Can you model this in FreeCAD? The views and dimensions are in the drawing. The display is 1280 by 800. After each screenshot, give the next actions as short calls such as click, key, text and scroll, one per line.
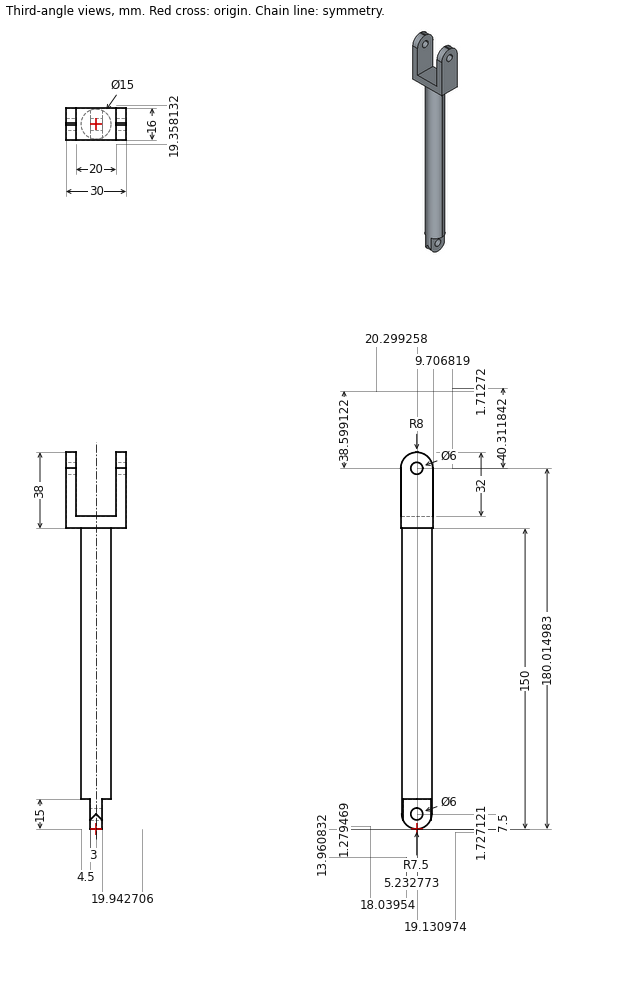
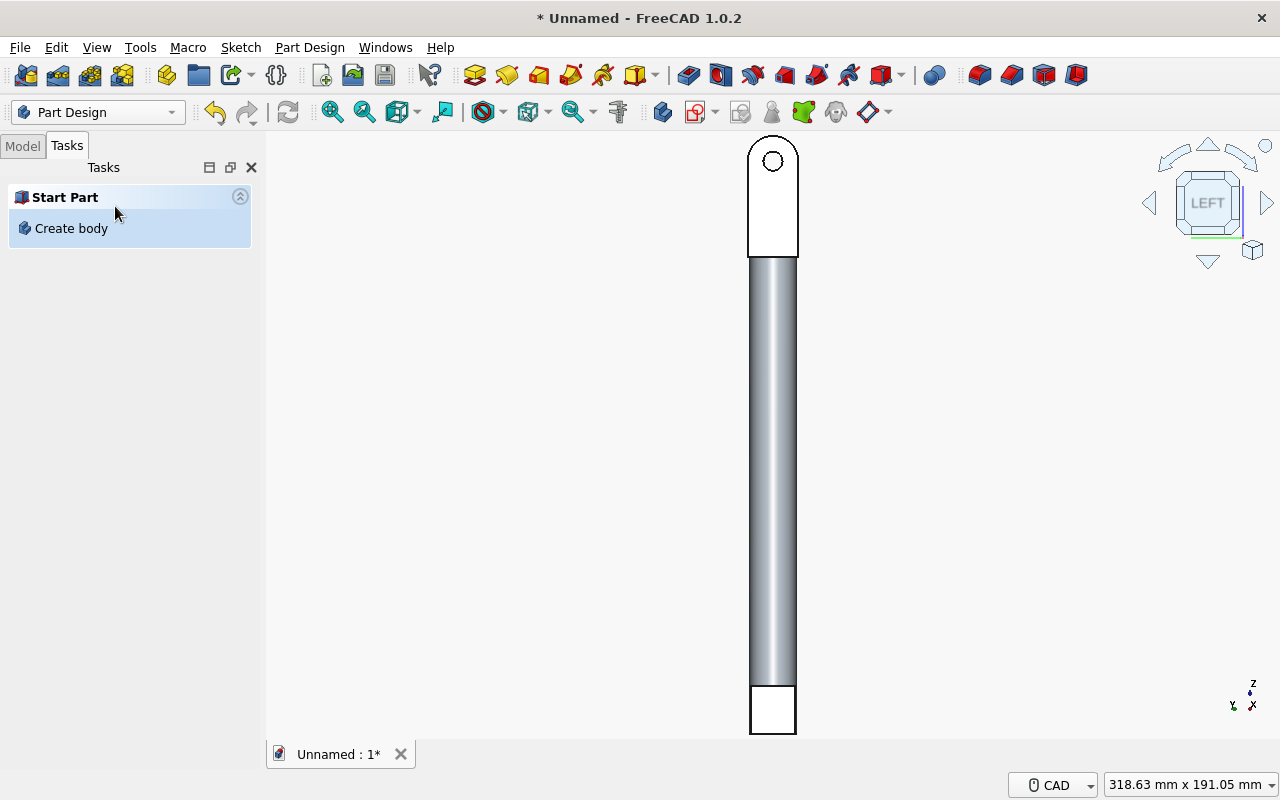
click(773, 709)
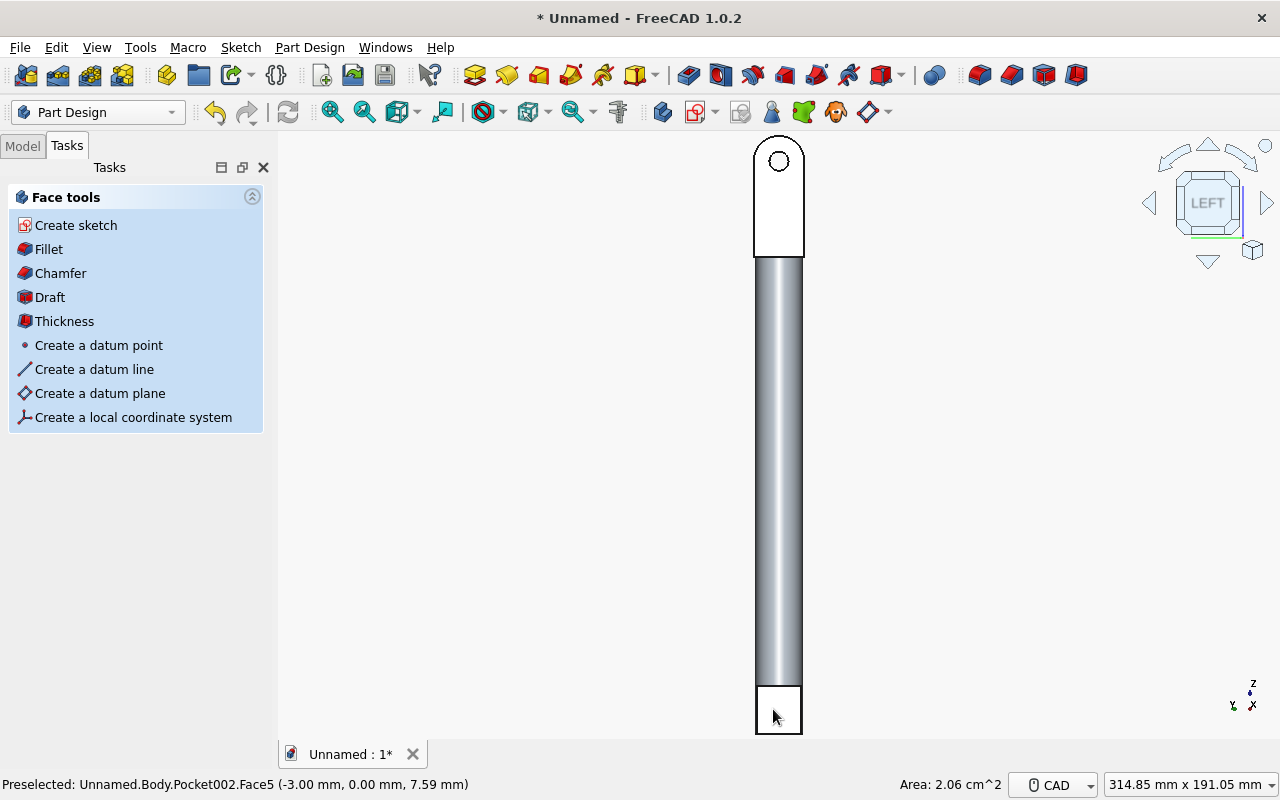
click(696, 112)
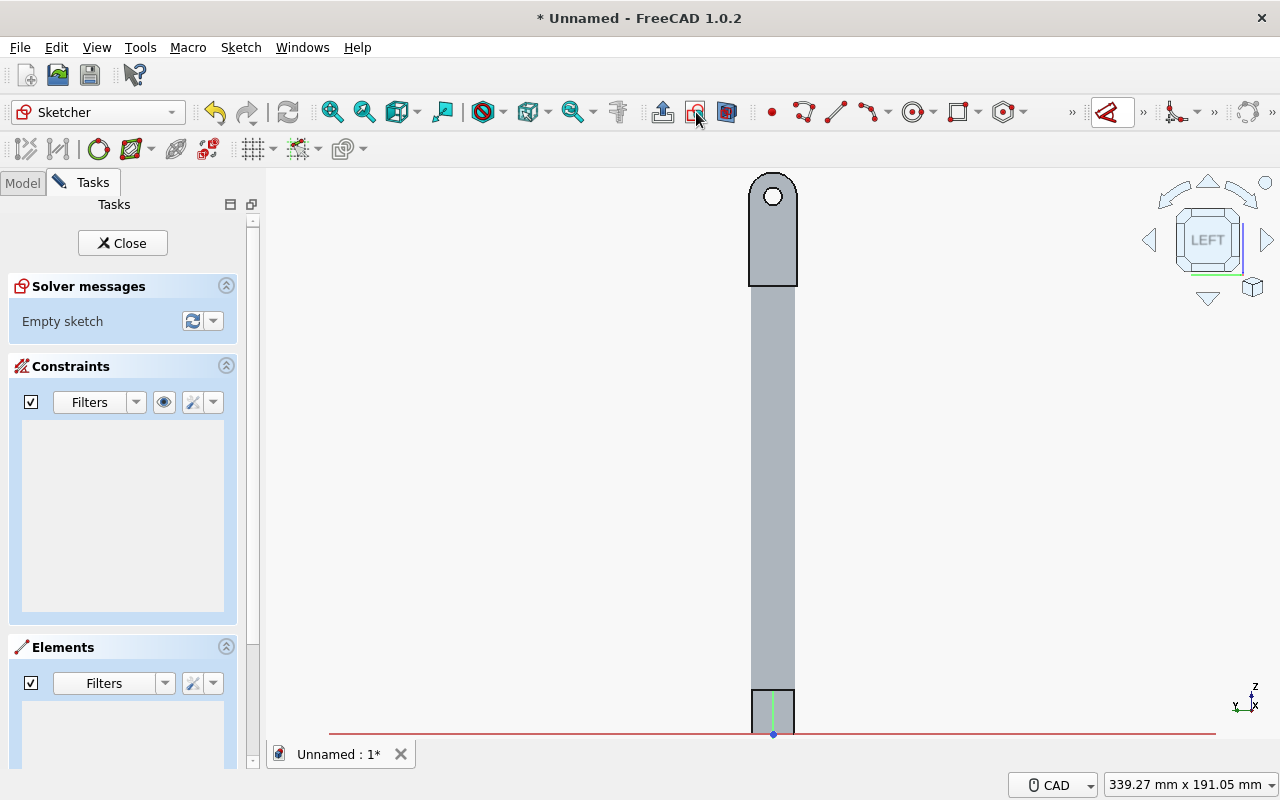
scroll(704, 454, down, 5)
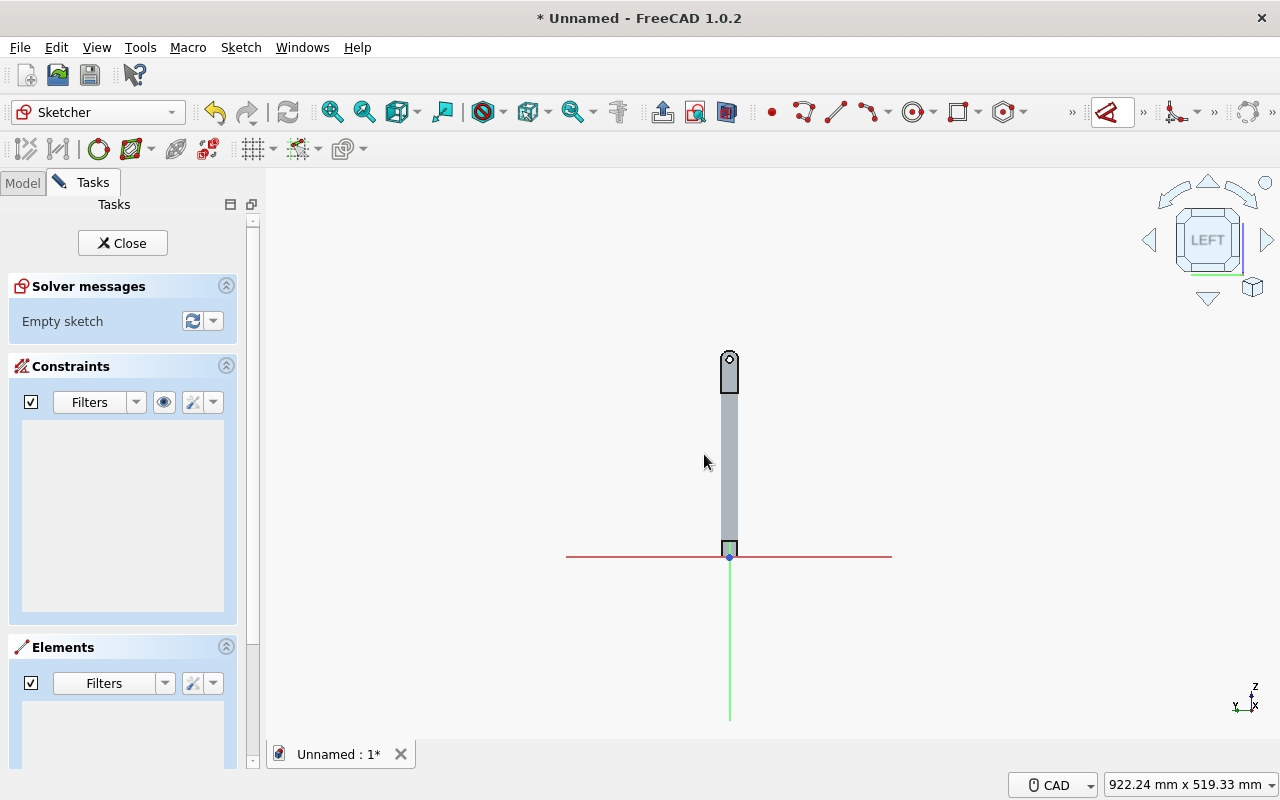
scroll(734, 568, up, 13)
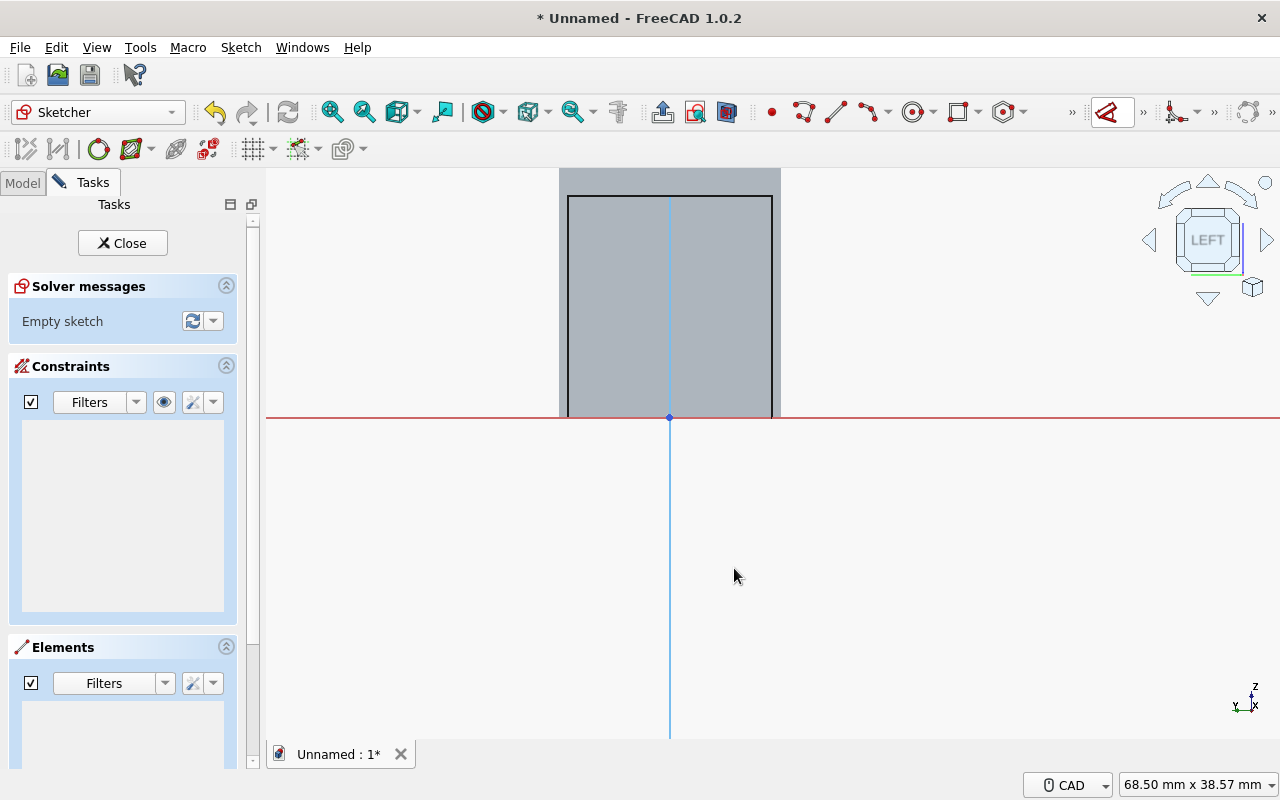
key(g)
key(m)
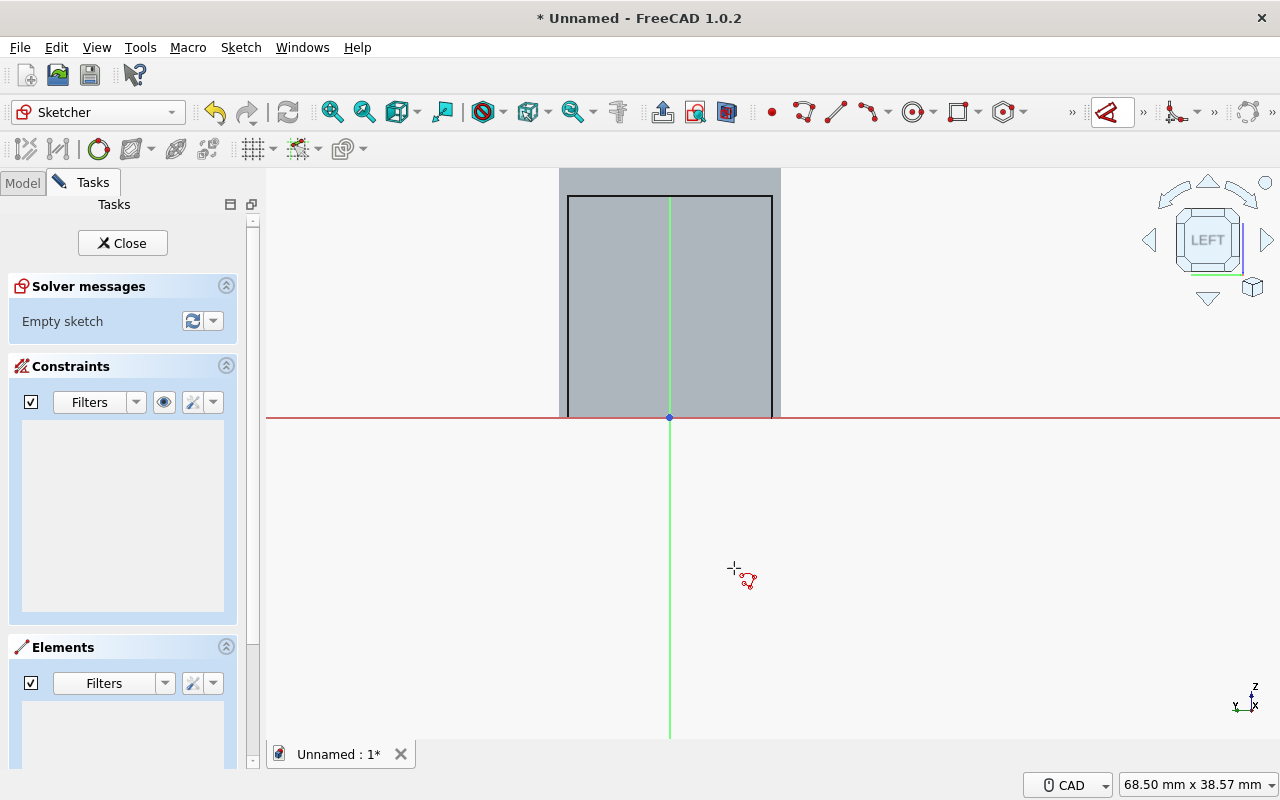
click(559, 307)
click(387, 443)
click(747, 624)
click(1014, 399)
click(781, 307)
right_click(781, 307)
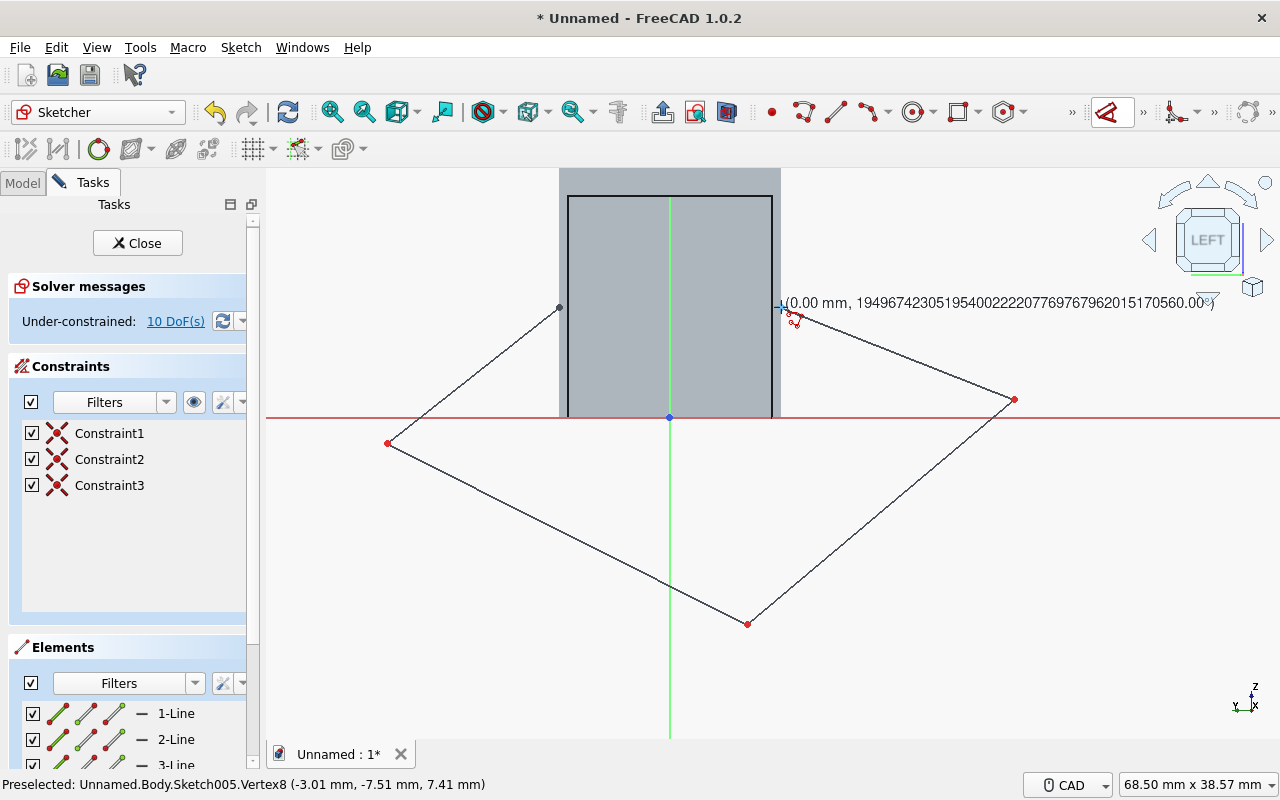
key(g)
key(3)
key(a)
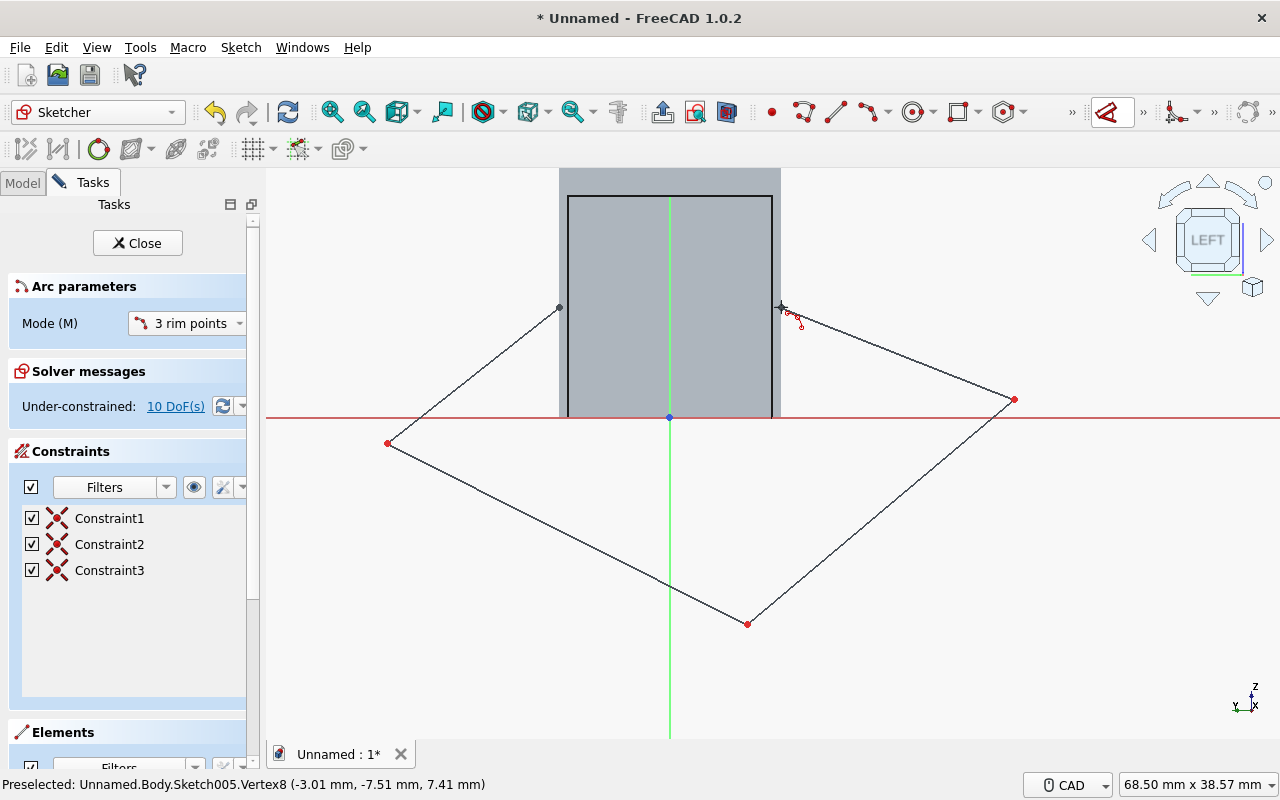
click(781, 308)
click(559, 308)
click(605, 396)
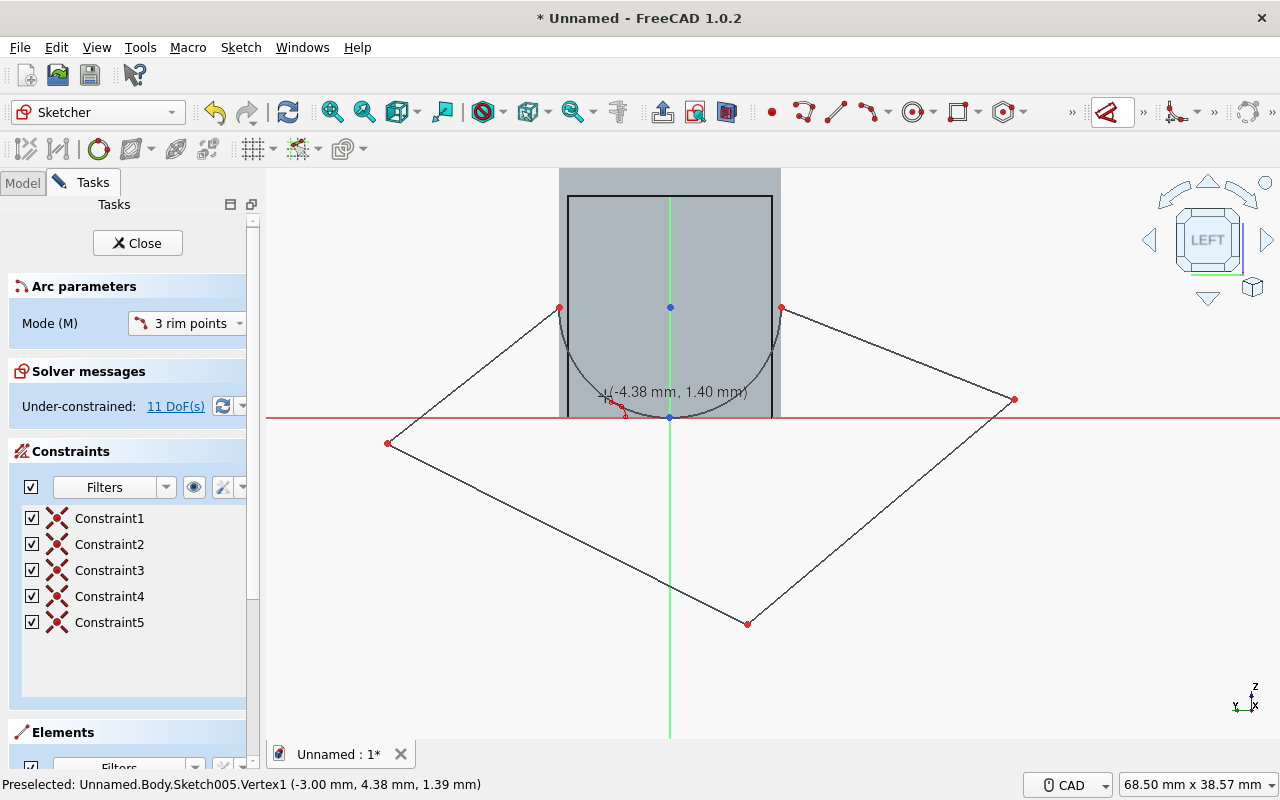
key(g)
key(c)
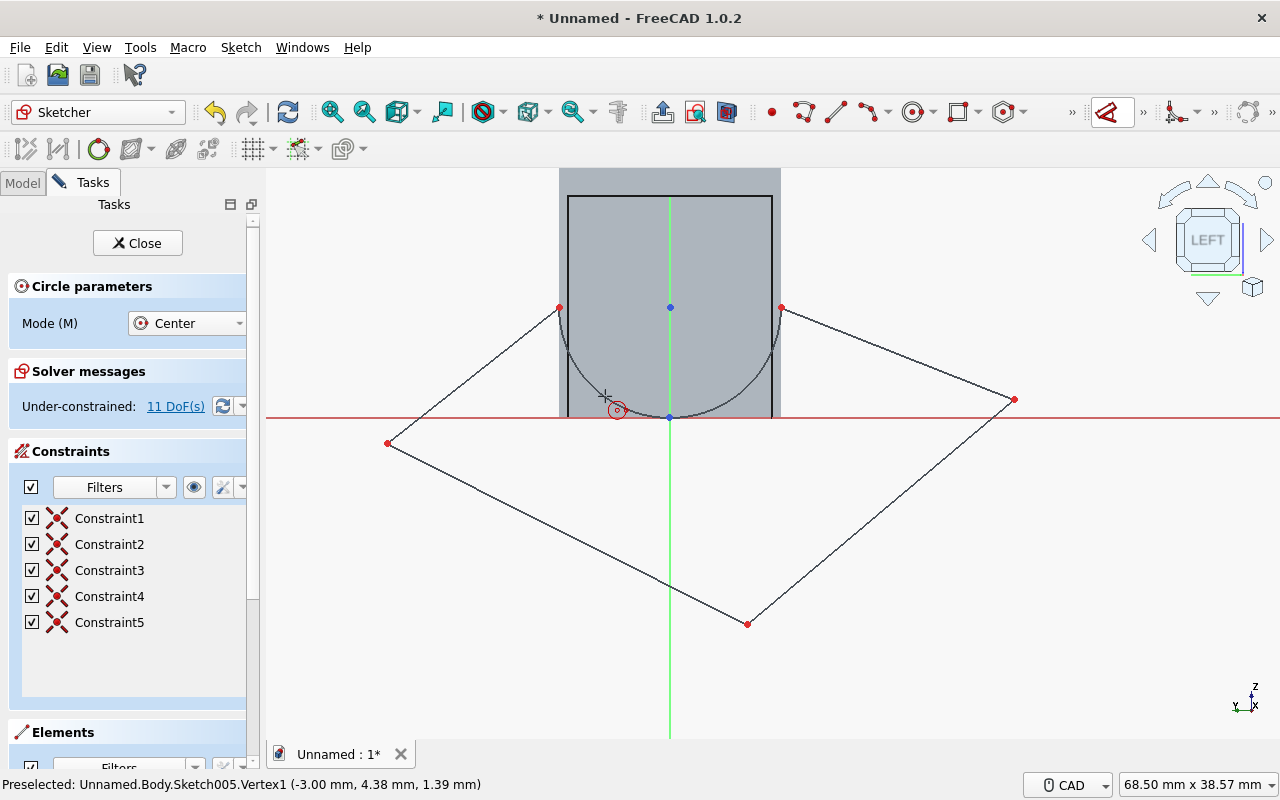
click(670, 307)
move(701, 275)